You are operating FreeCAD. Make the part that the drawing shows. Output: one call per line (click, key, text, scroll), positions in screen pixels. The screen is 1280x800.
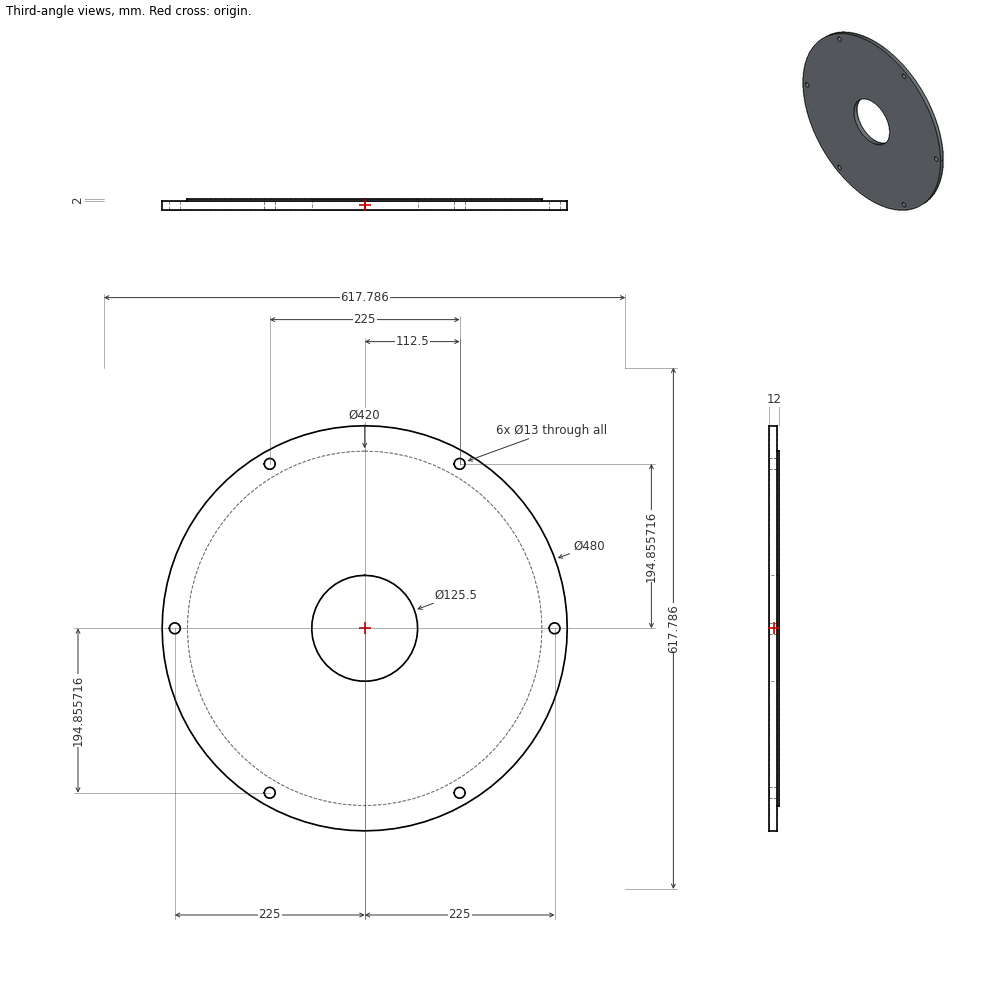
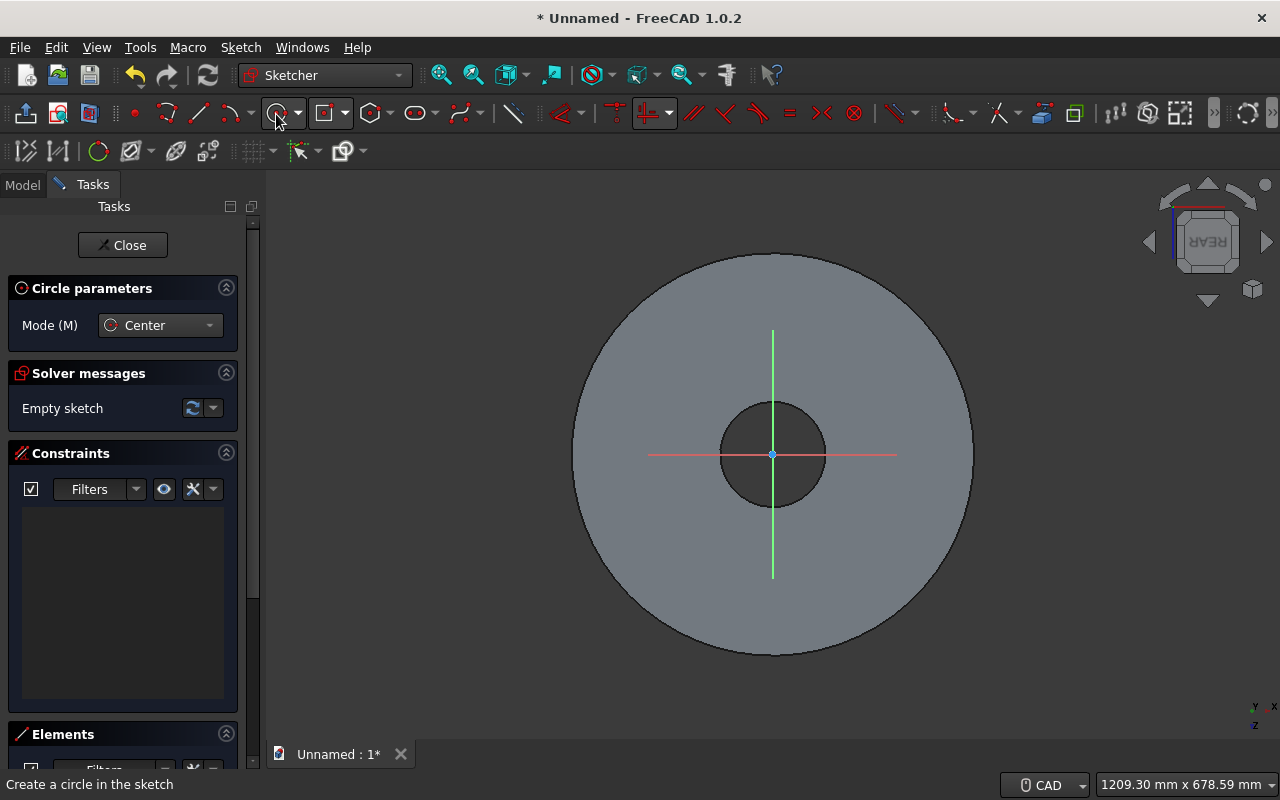
scroll(867, 618, up, 8)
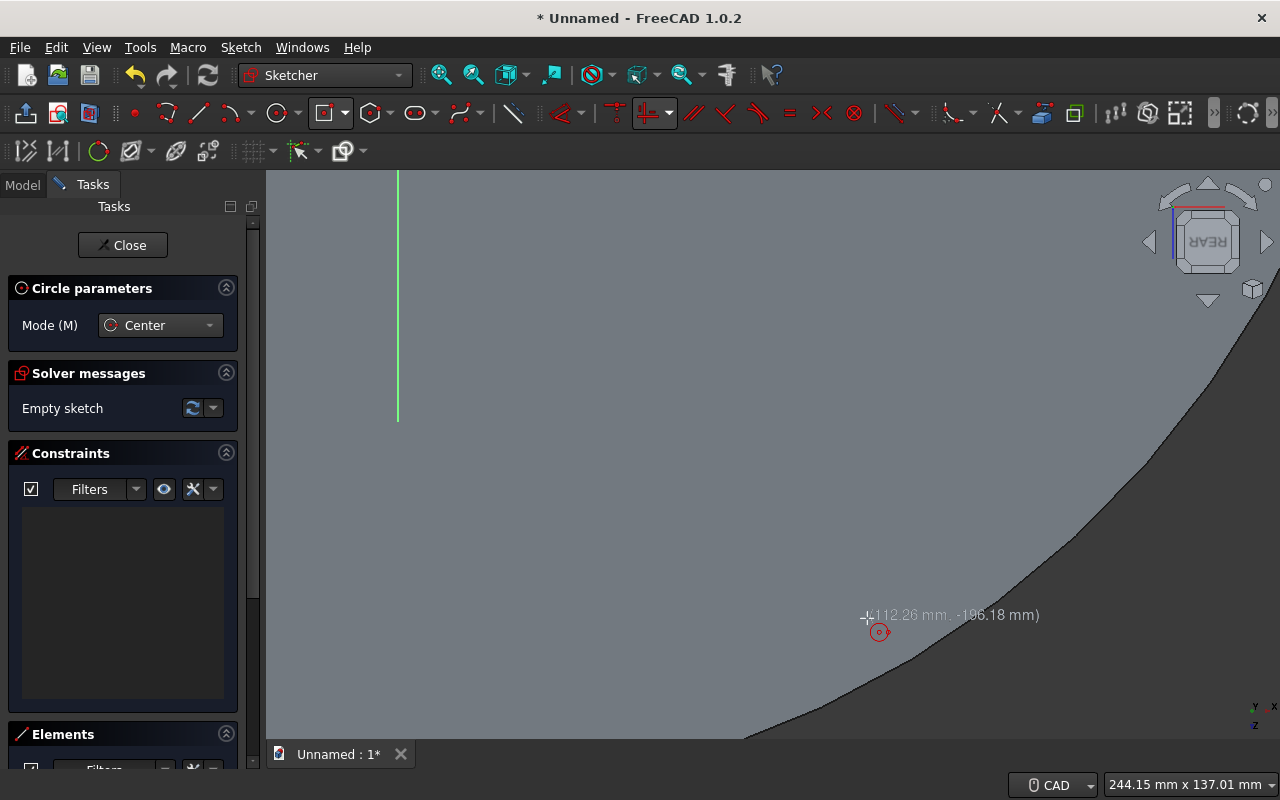
scroll(782, 619, down, 8)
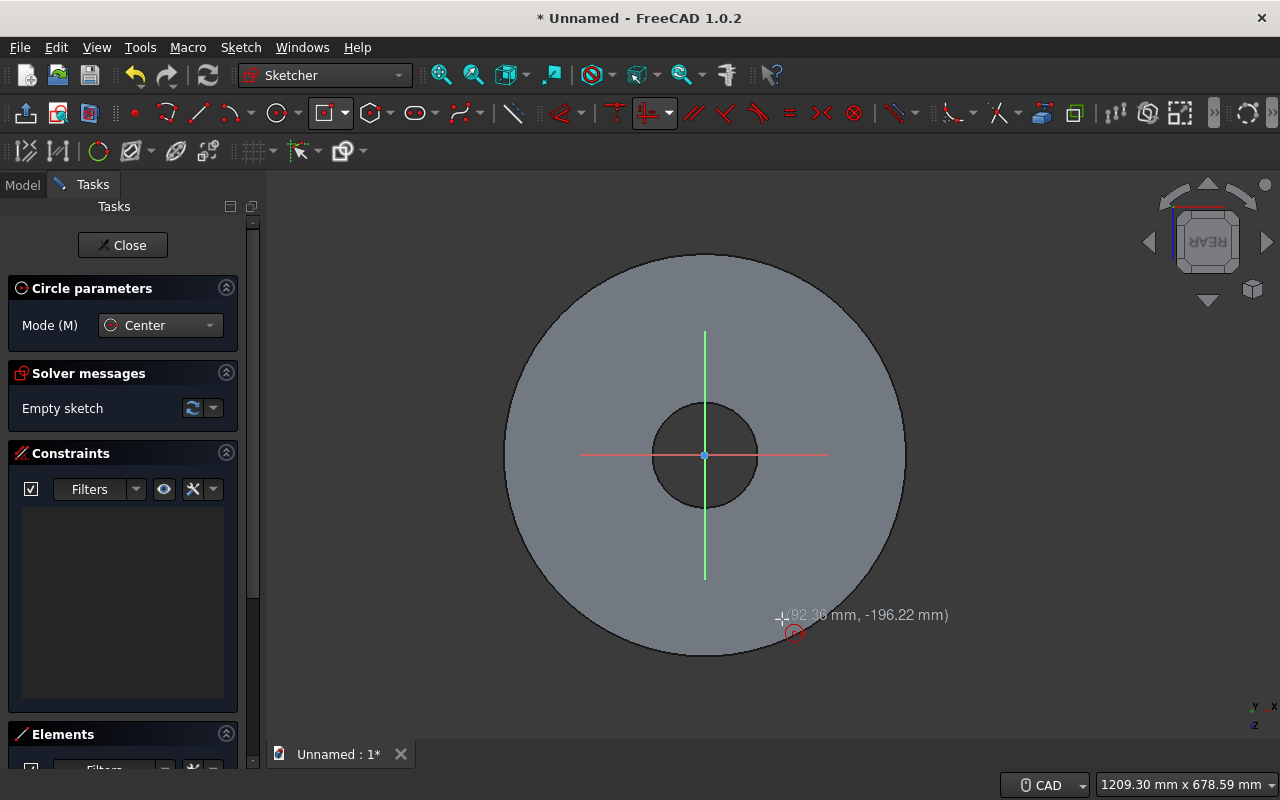
click(799, 619)
move(803, 615)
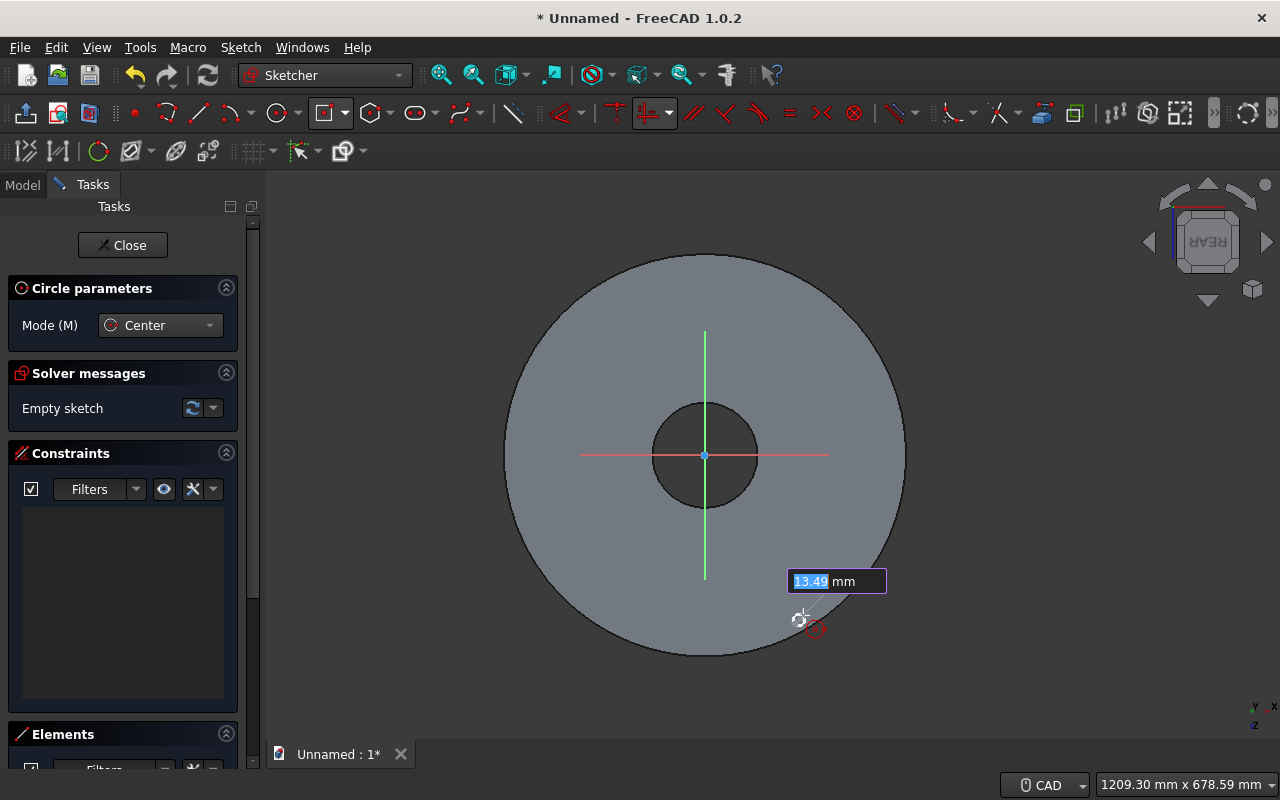
text(13)
key(Return)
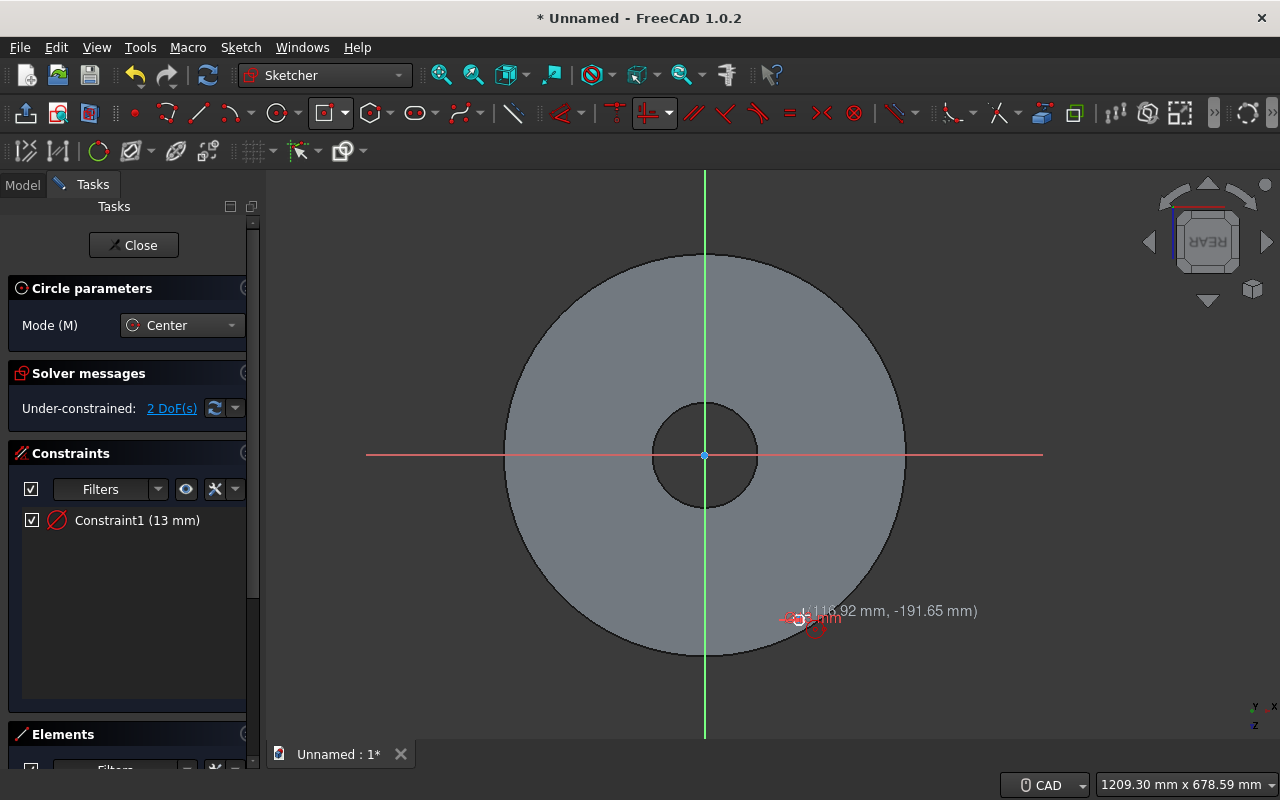
scroll(611, 619, up, 8)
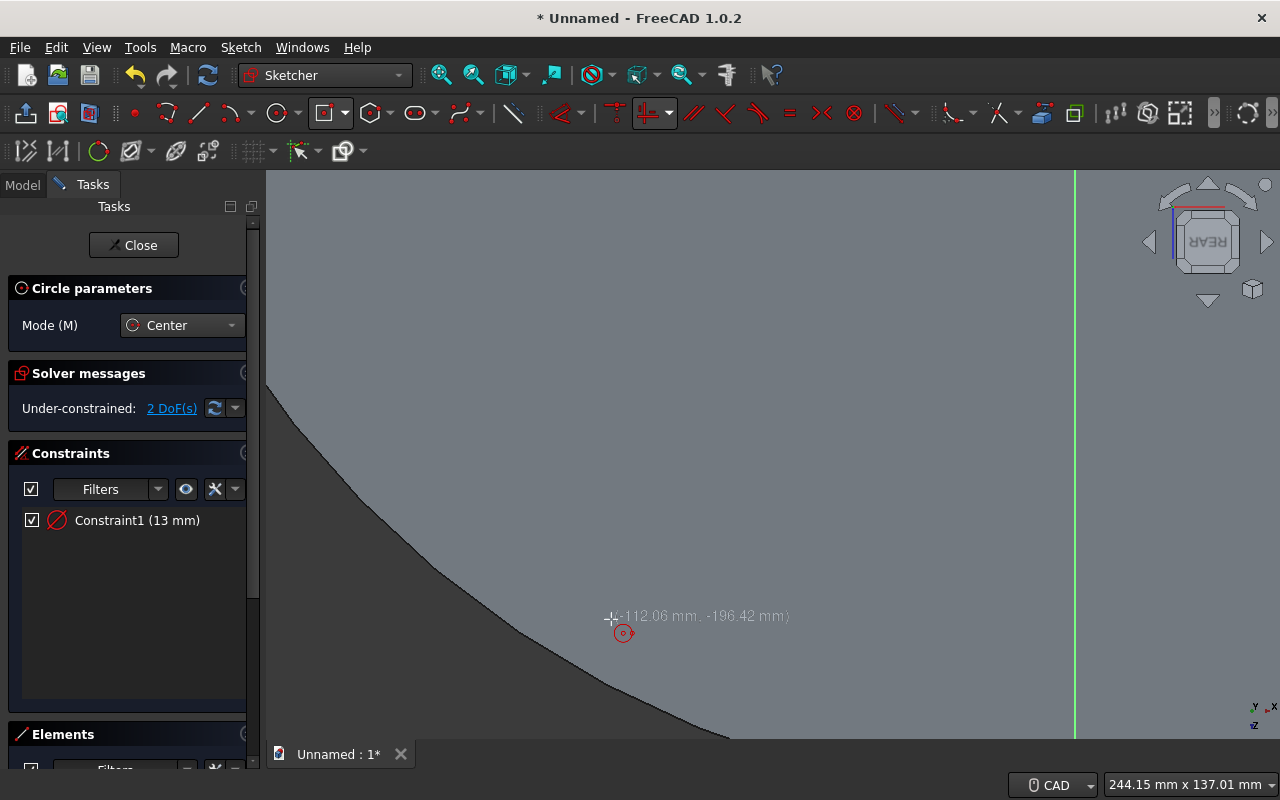
scroll(611, 619, down, 8)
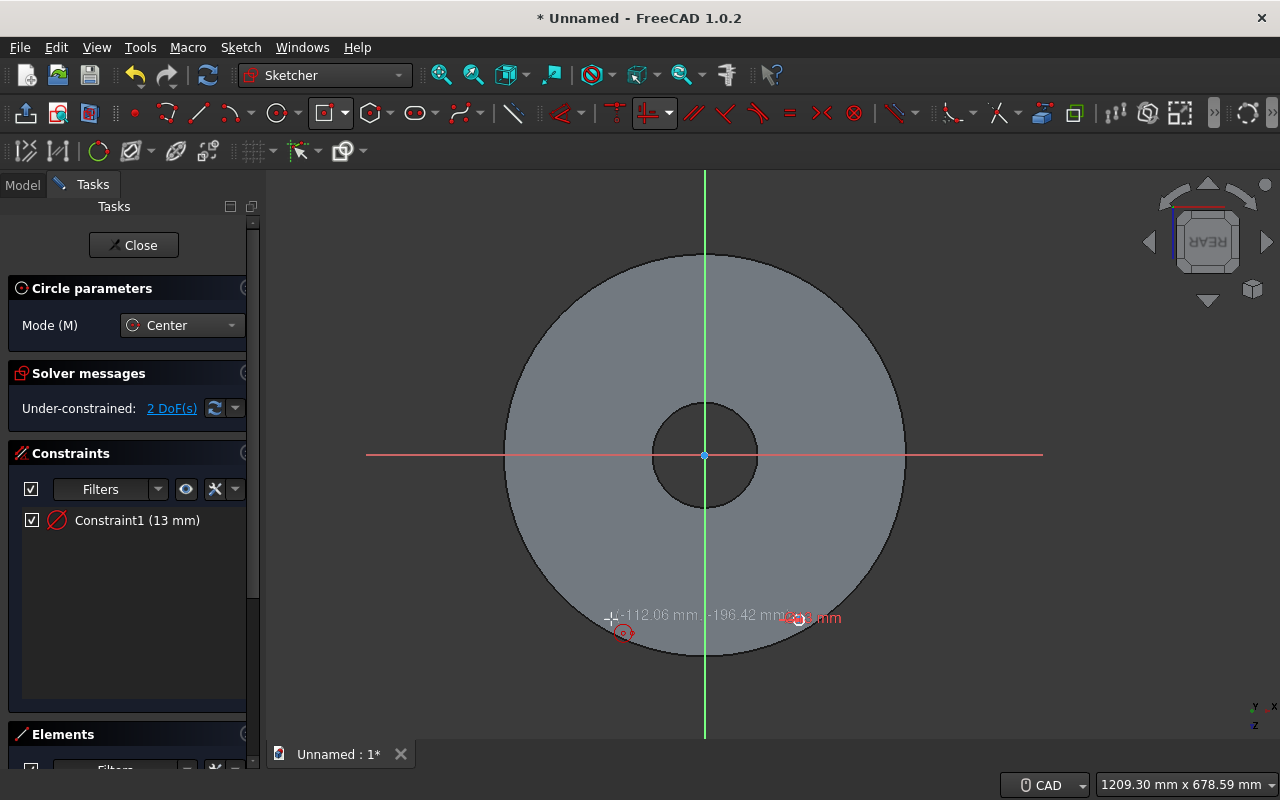
click(611, 619)
move(614, 615)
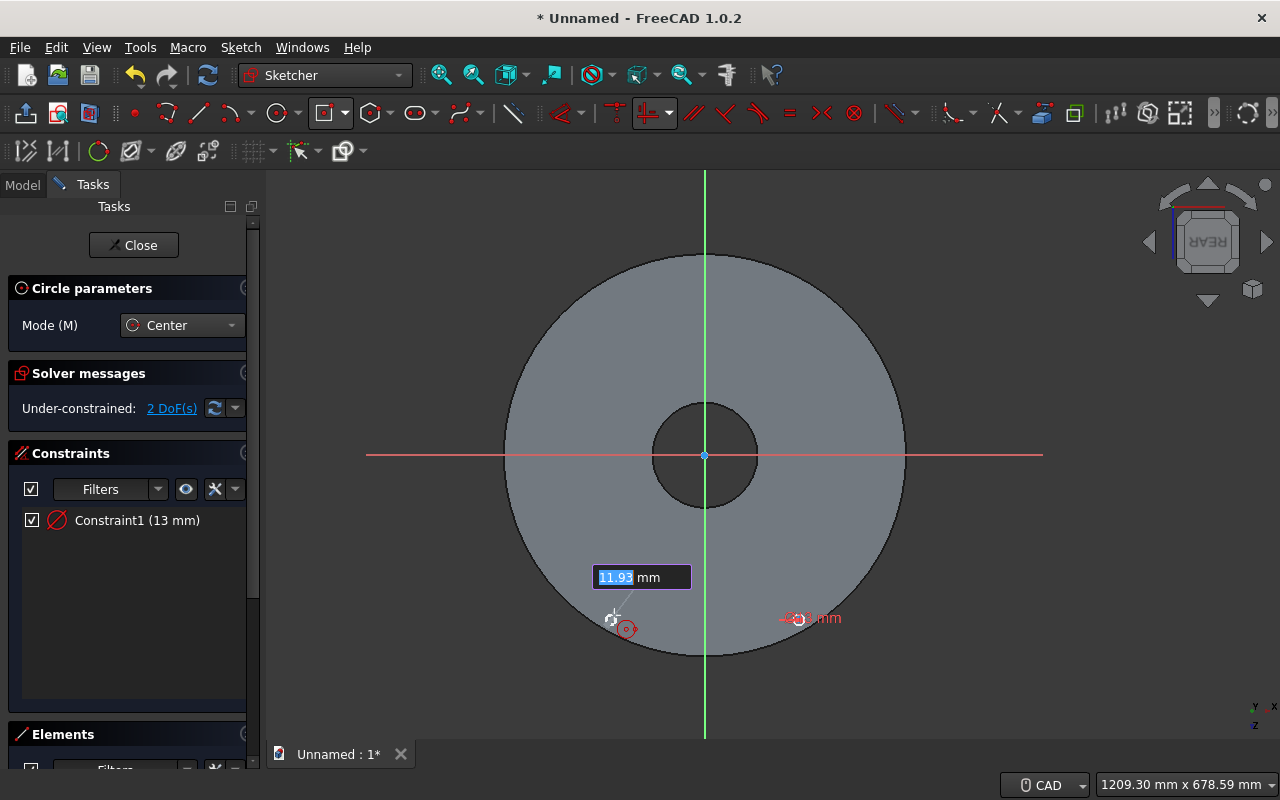
text(13)
key(Return)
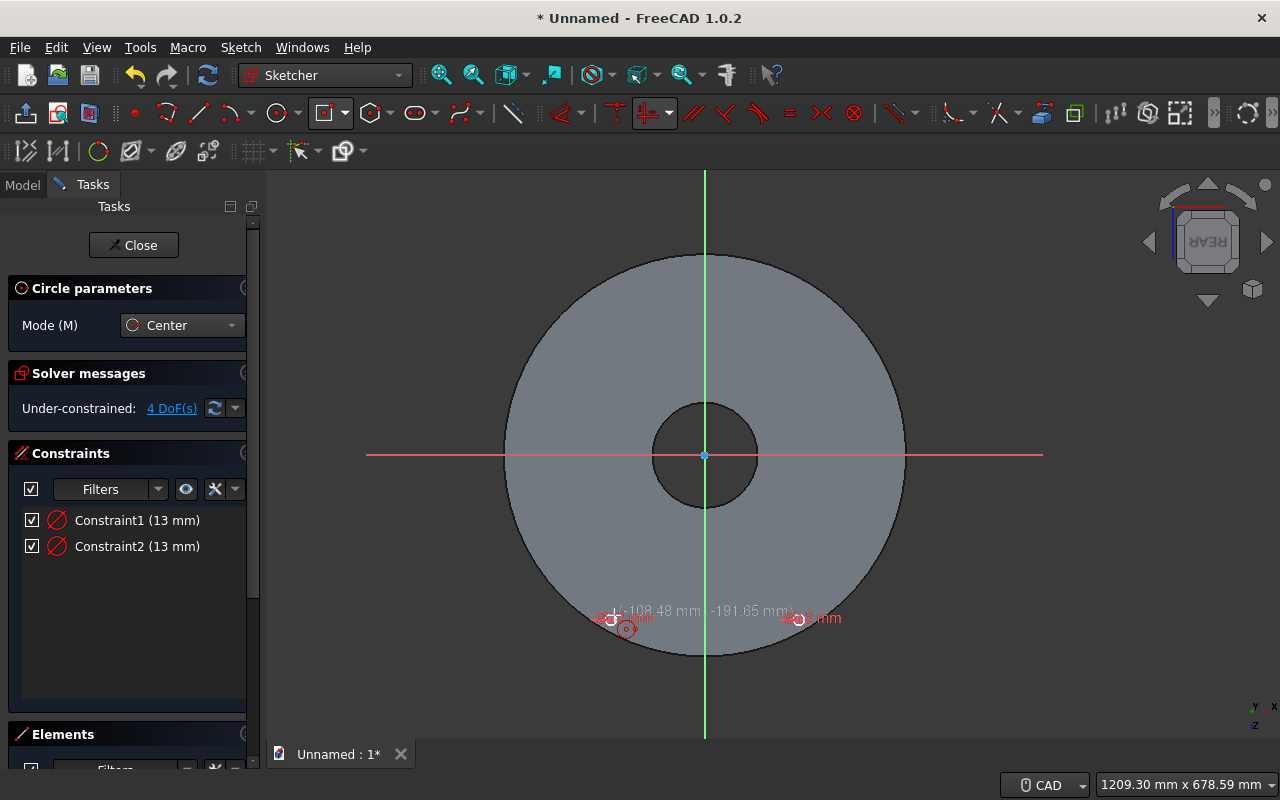
scroll(516, 455, up, 8)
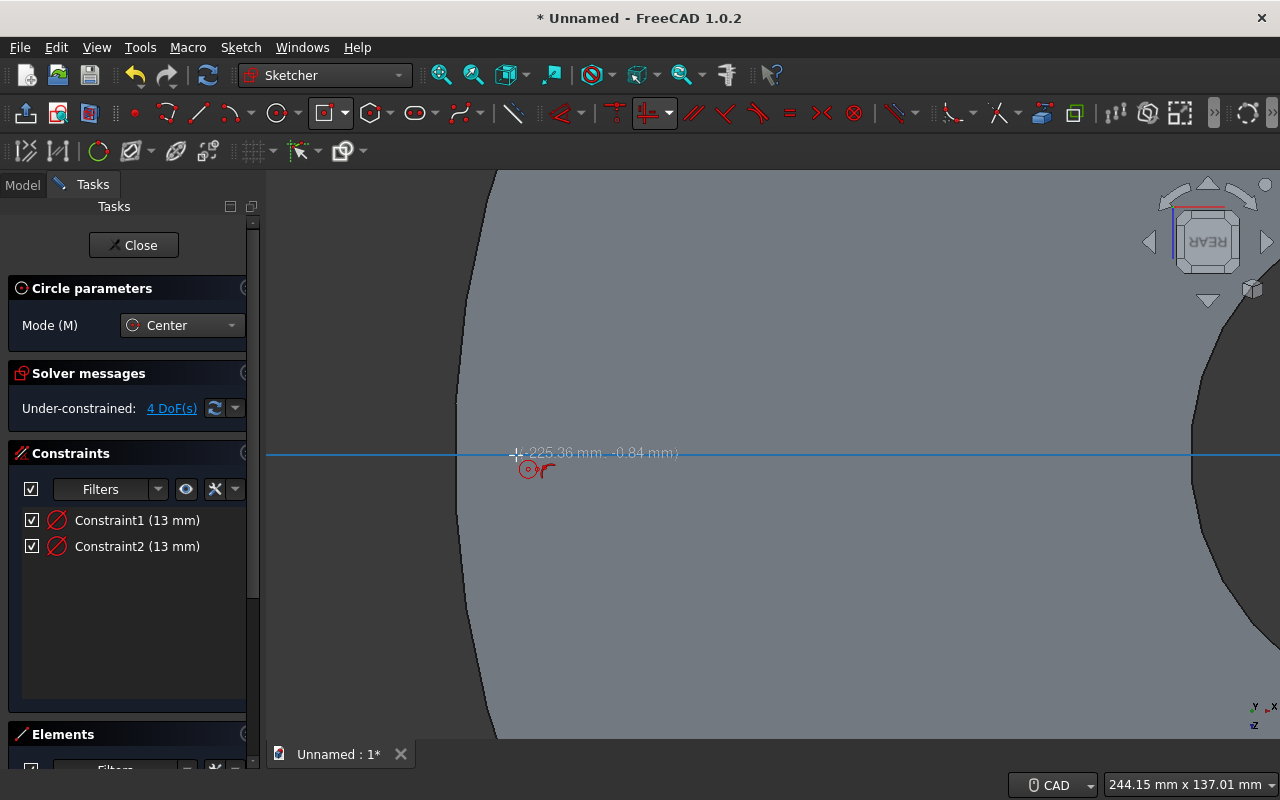
scroll(516, 454, down, 8)